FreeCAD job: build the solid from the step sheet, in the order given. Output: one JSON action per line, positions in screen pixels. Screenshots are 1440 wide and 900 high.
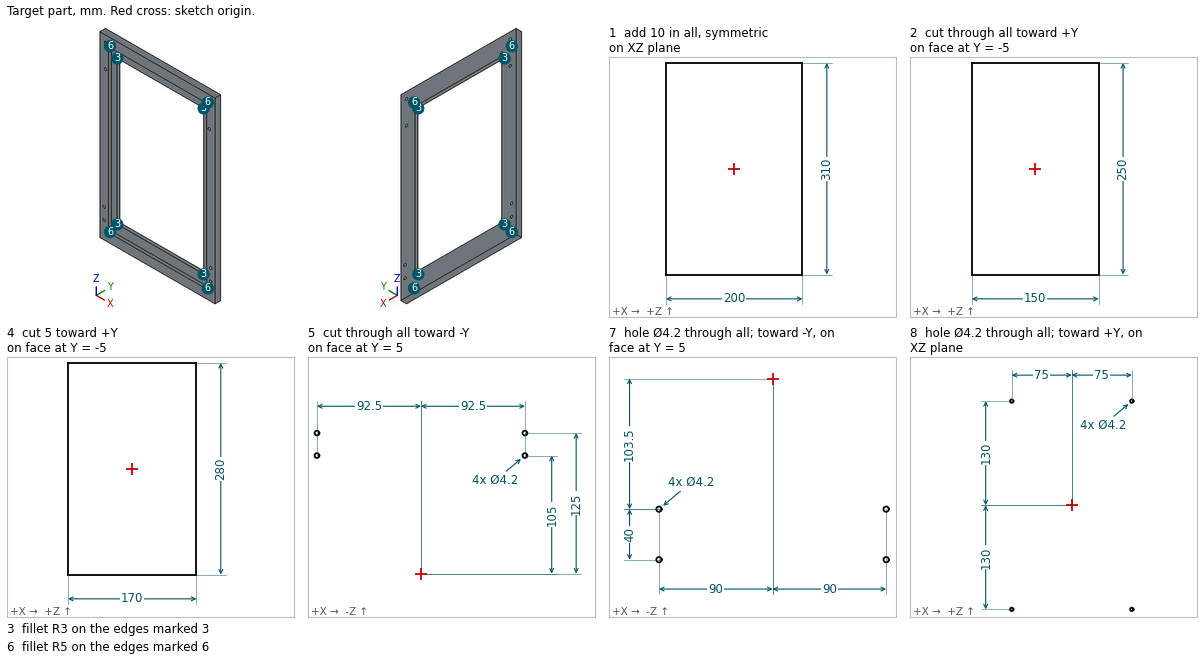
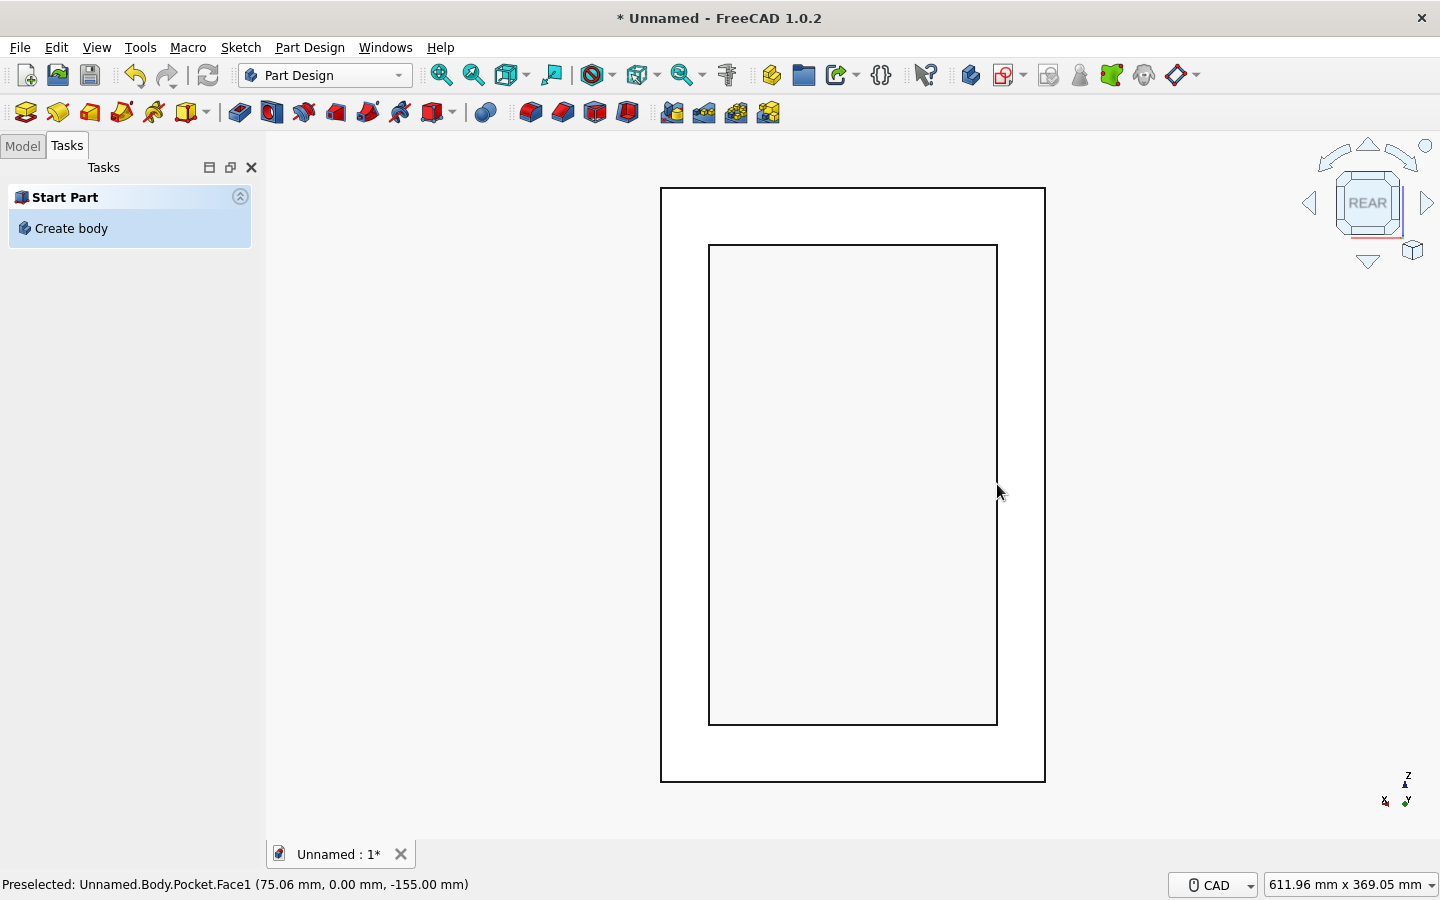
{"action": "scroll", "coordinate": [709, 244], "scroll_direction": "up", "scroll_amount": 4}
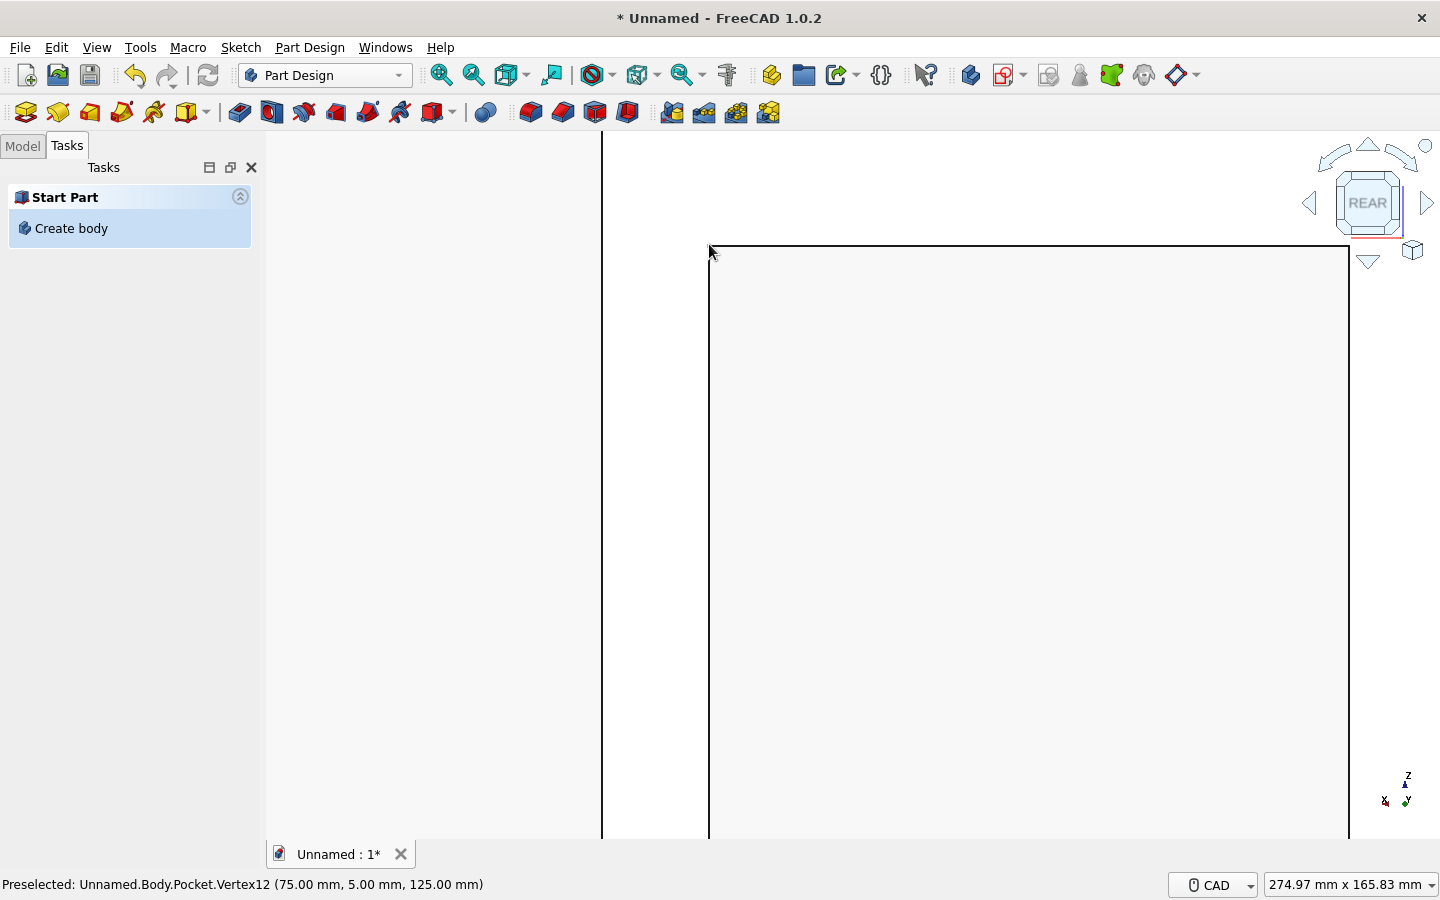
{"action": "key", "text": "v f"}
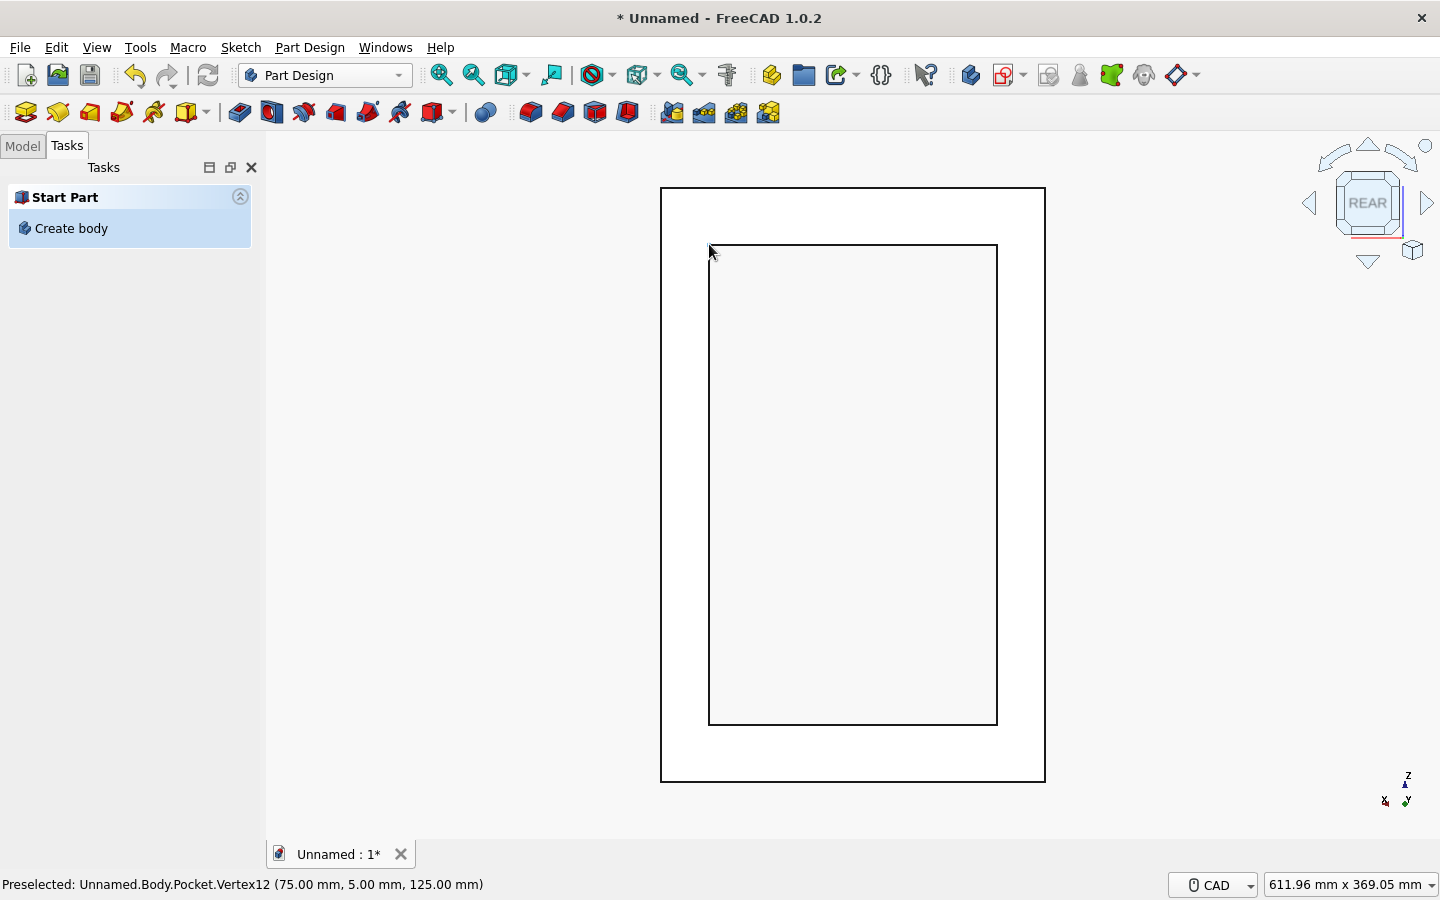
{"action": "key", "text": "6"}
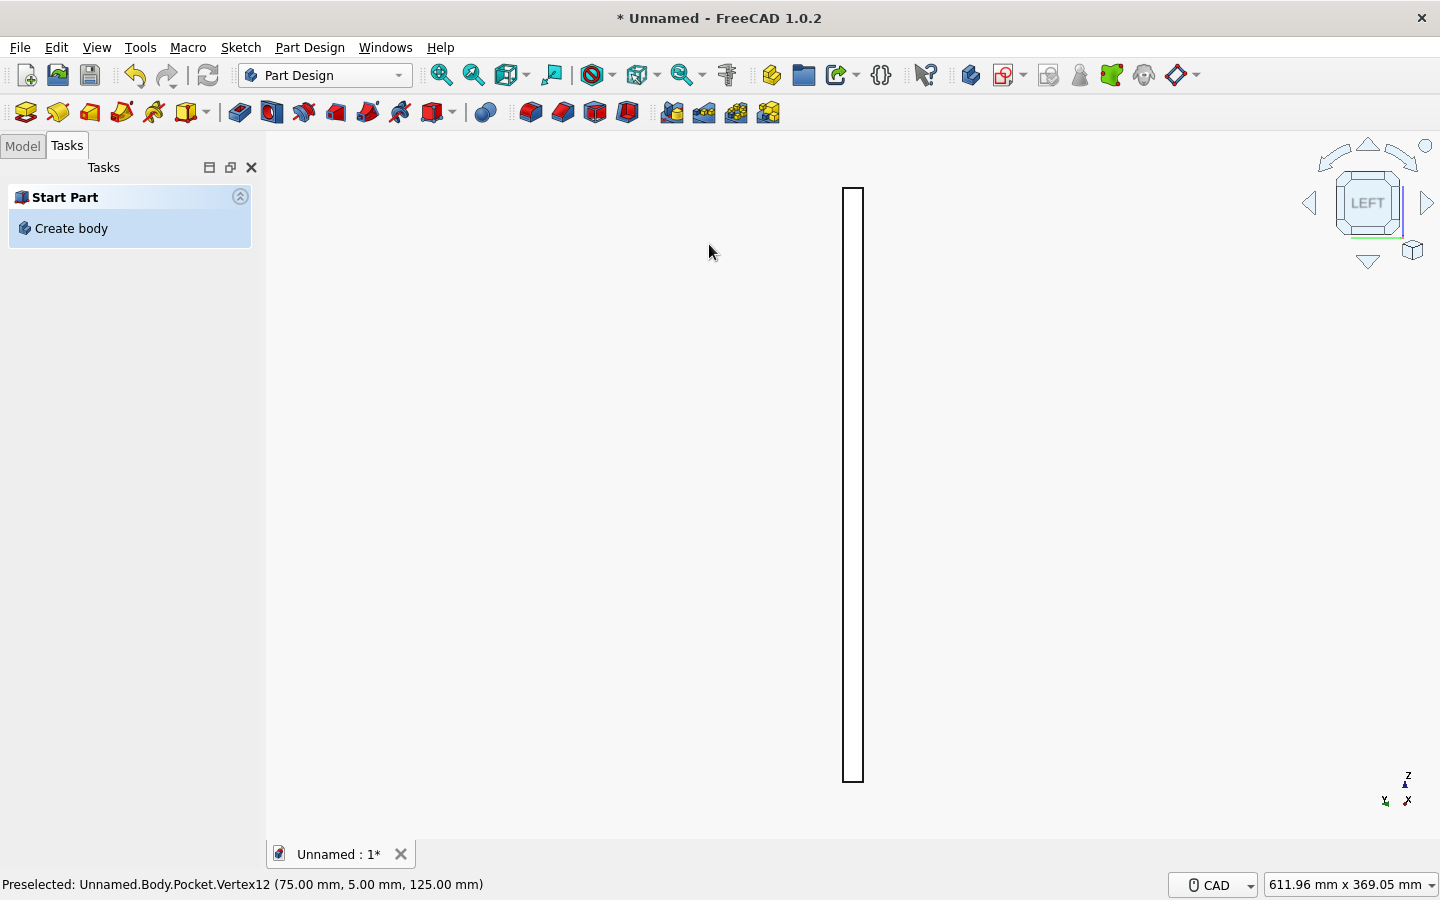
{"action": "scroll", "coordinate": [853, 244], "scroll_direction": "up", "scroll_amount": 4}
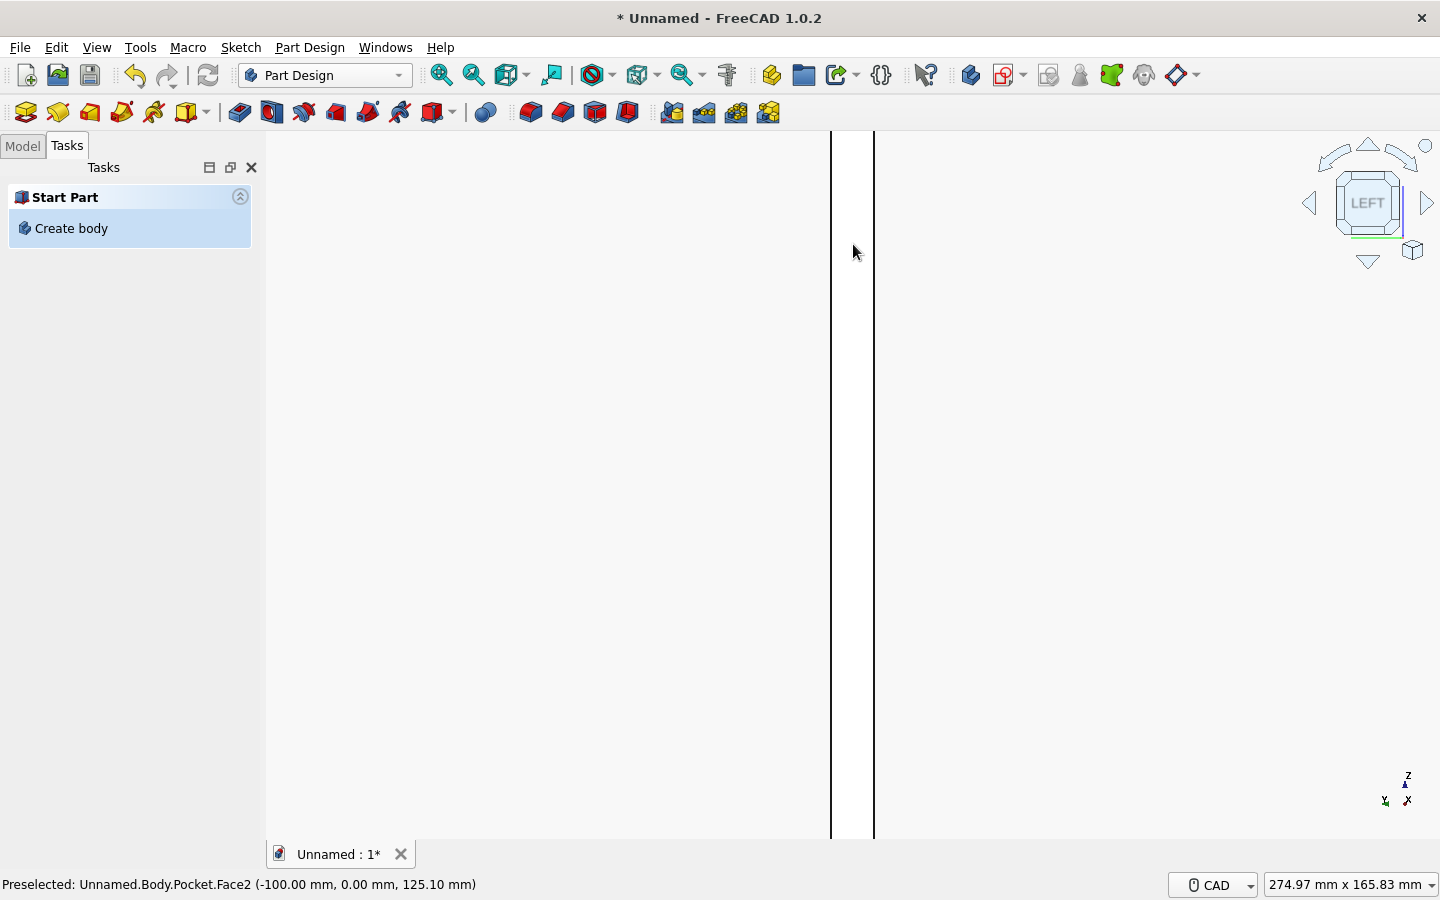
{"action": "key", "text": "v f"}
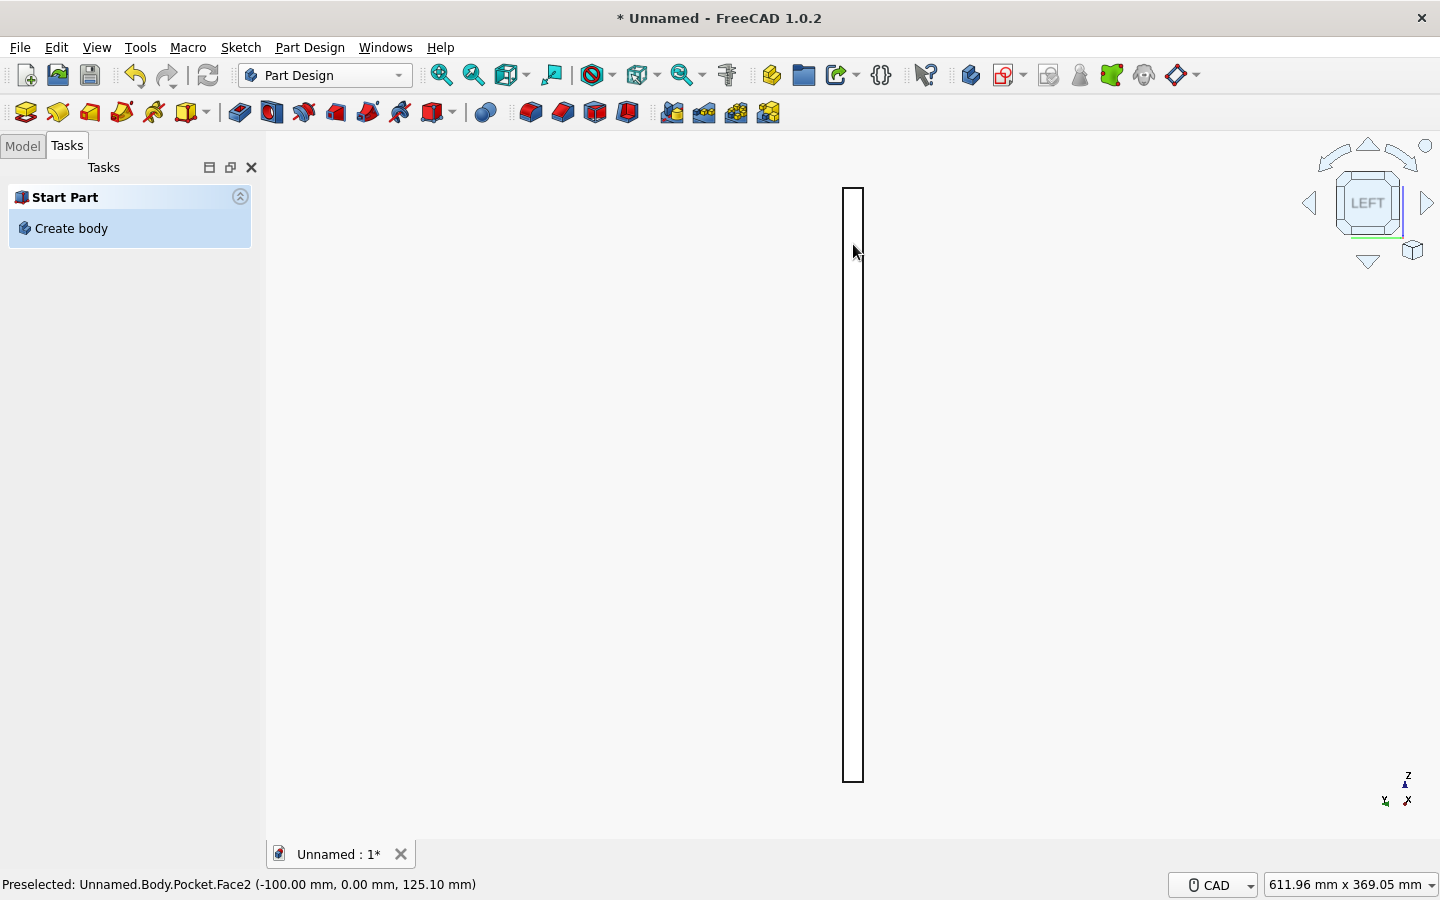
{"action": "key", "text": "v 3"}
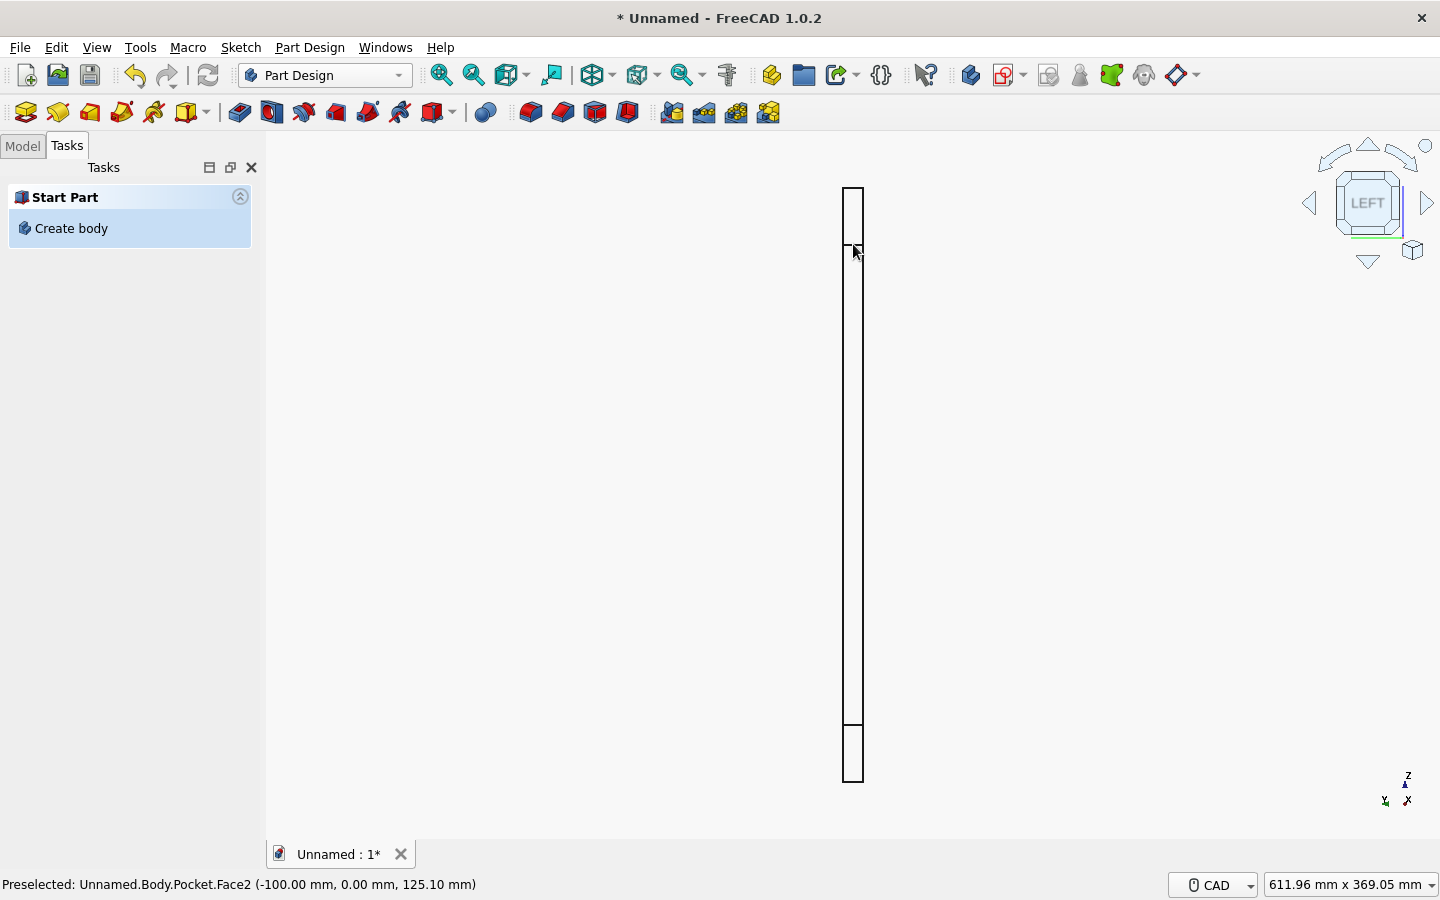
{"action": "key", "text": "0"}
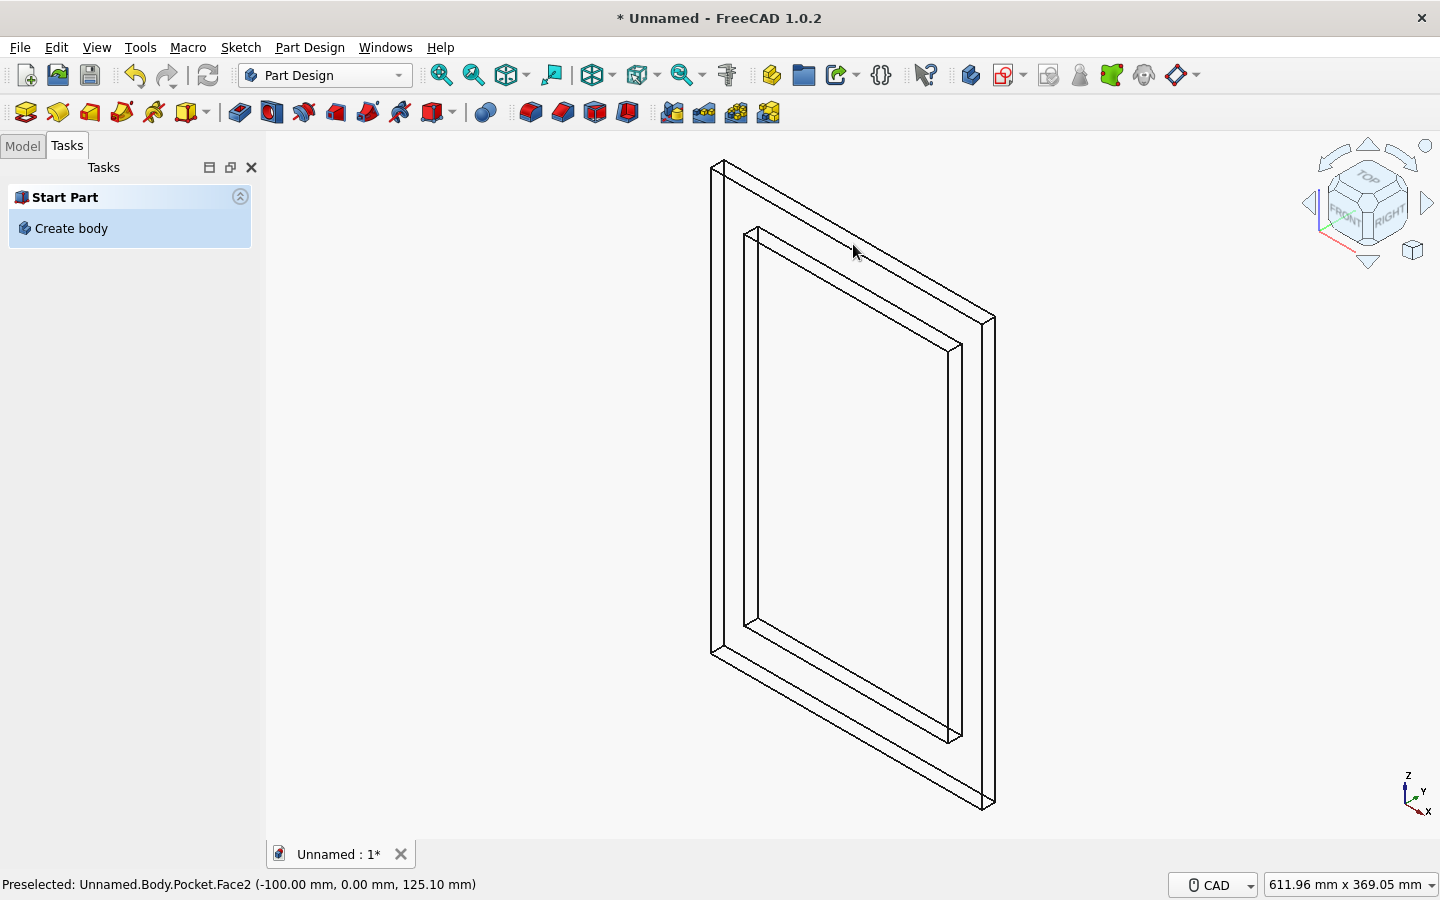
{"action": "left_click", "coordinate": [955, 347]}